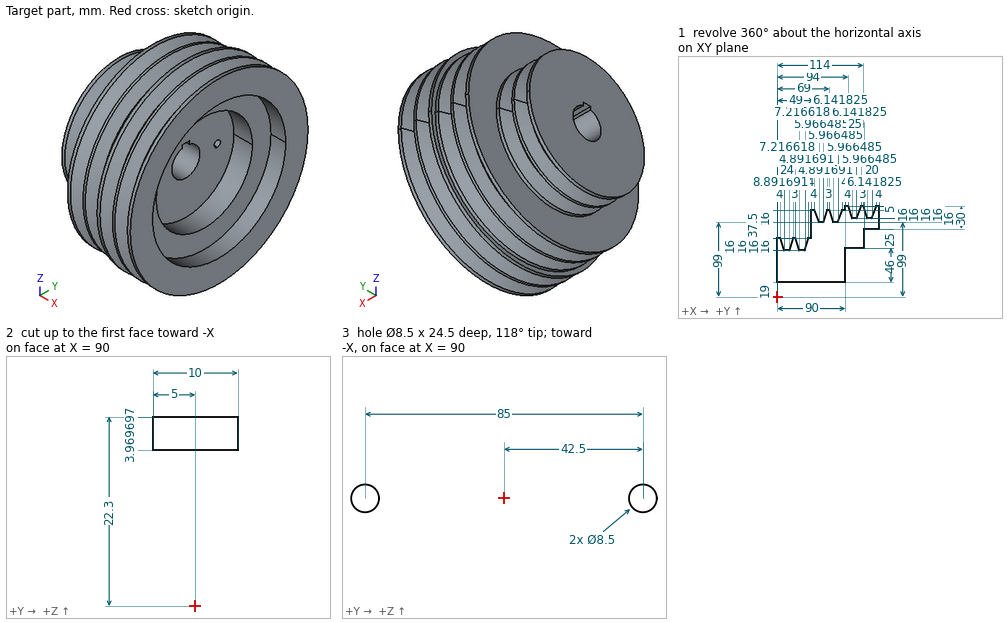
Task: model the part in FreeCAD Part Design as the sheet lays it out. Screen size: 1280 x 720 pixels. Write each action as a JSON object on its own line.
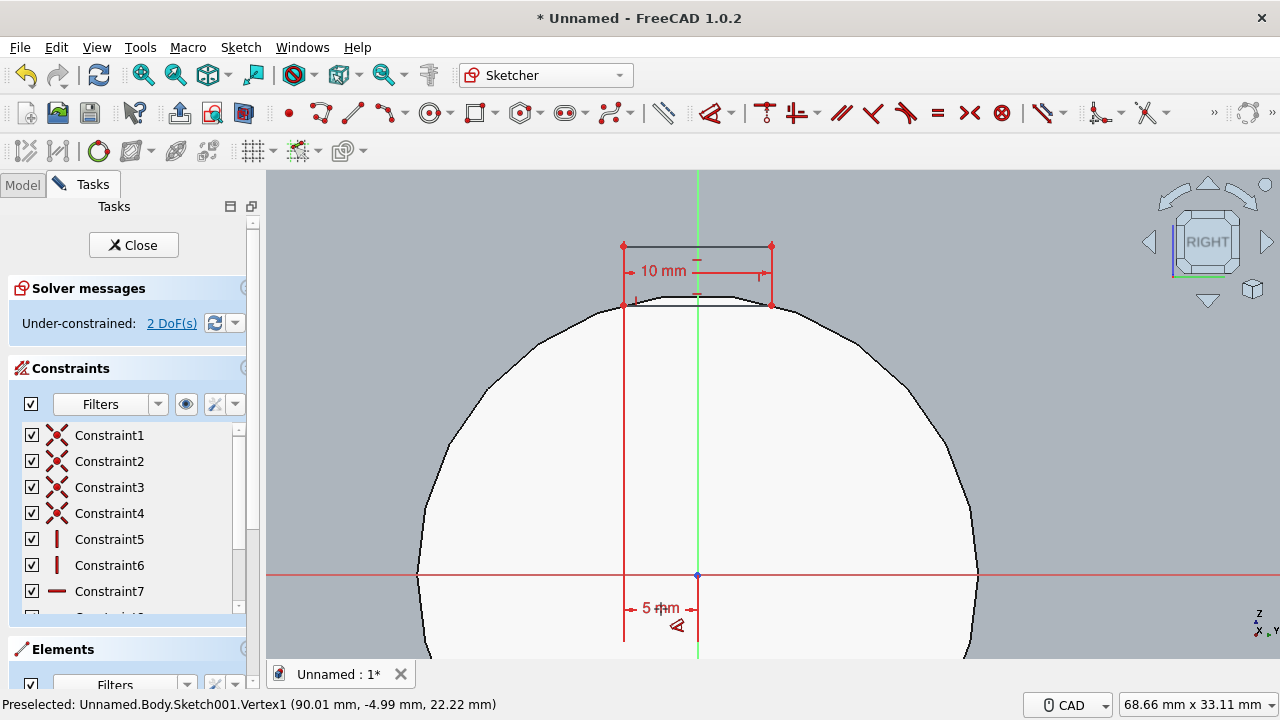
{"action": "left_click", "coordinate": [624, 247]}
{"action": "left_click", "coordinate": [590, 411]}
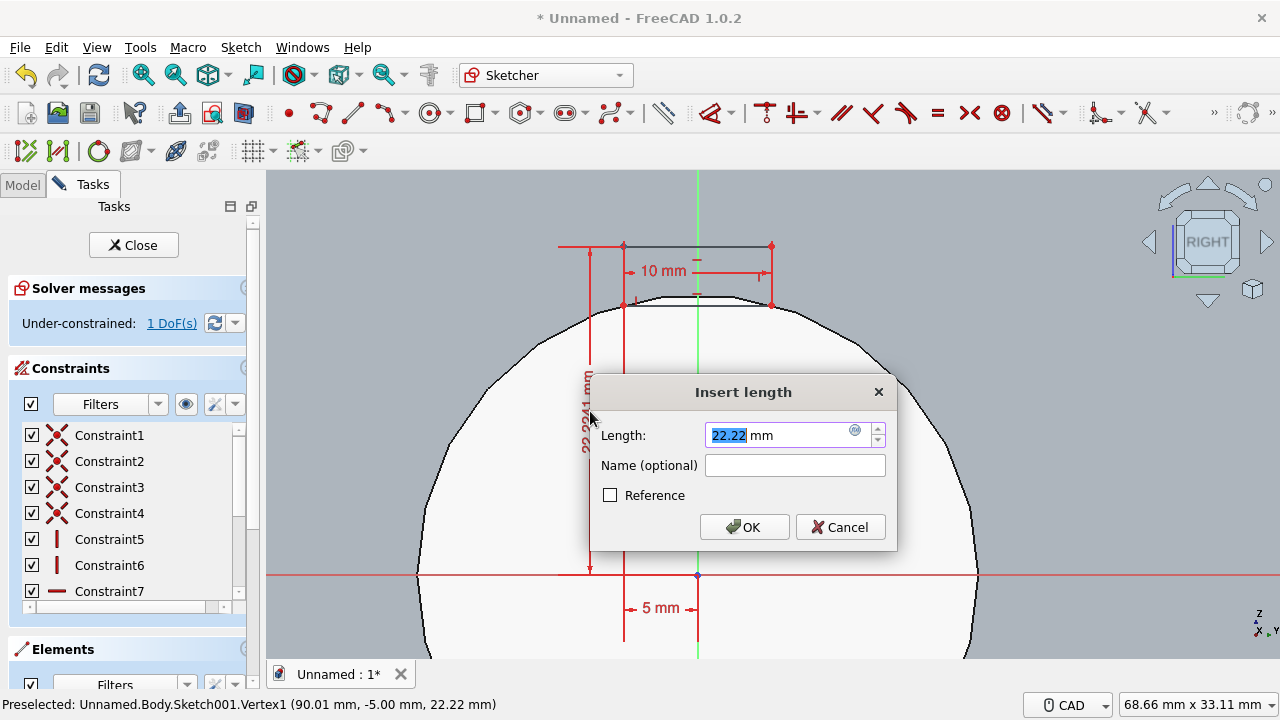
{"action": "type", "text": "22.3"}
{"action": "key", "text": "Return"}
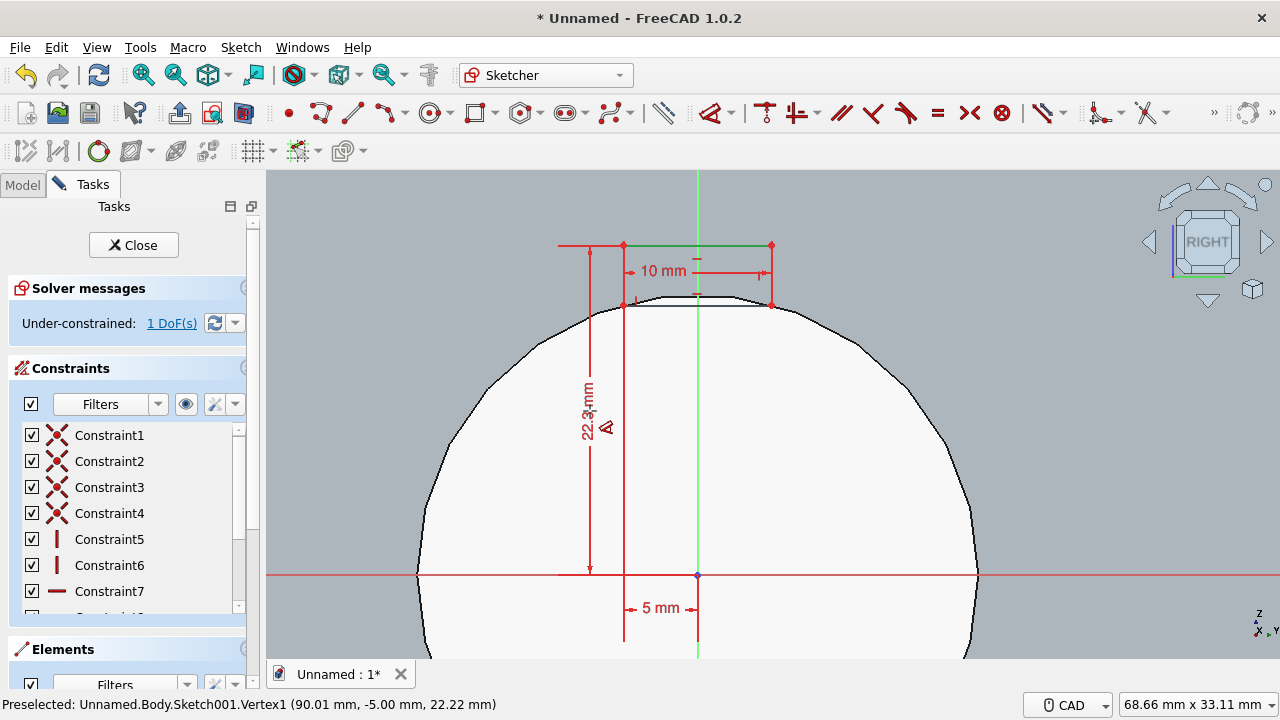
{"action": "left_click", "coordinate": [624, 264]}
{"action": "left_click", "coordinate": [590, 276]}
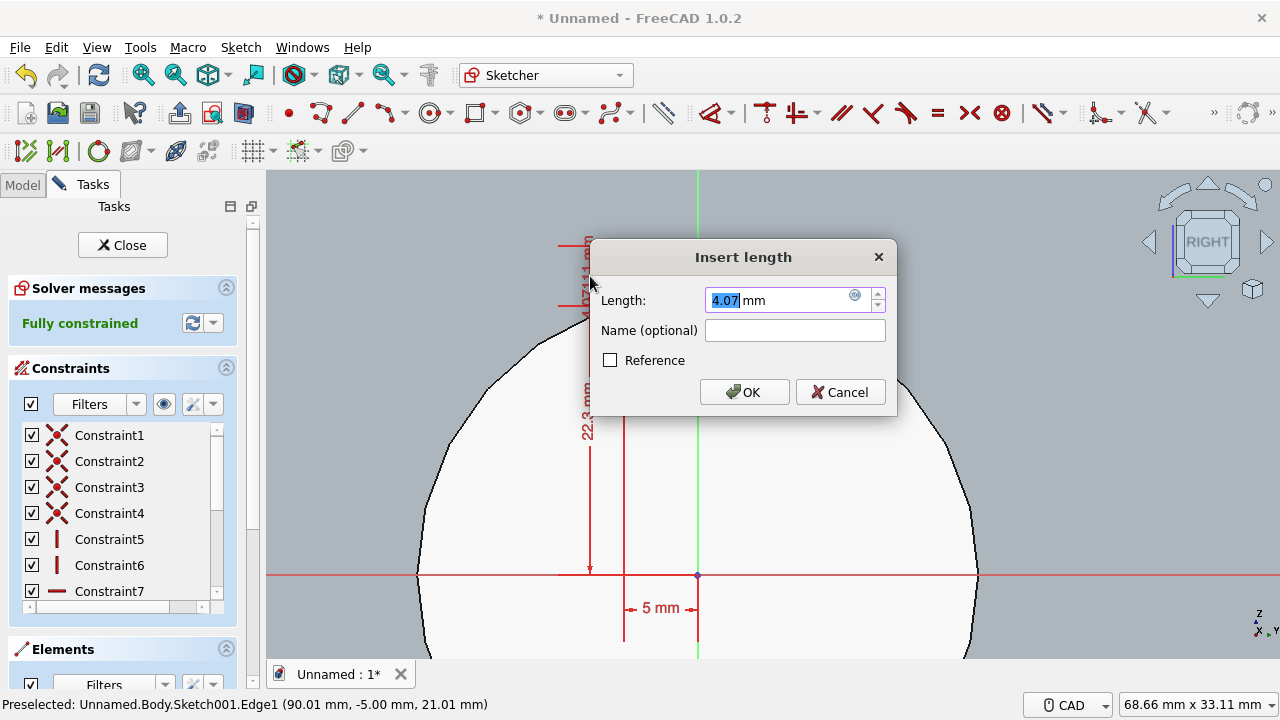
{"action": "type", "text": "3.969697"}
{"action": "key", "text": "Return"}
{"action": "key", "text": "Escape"}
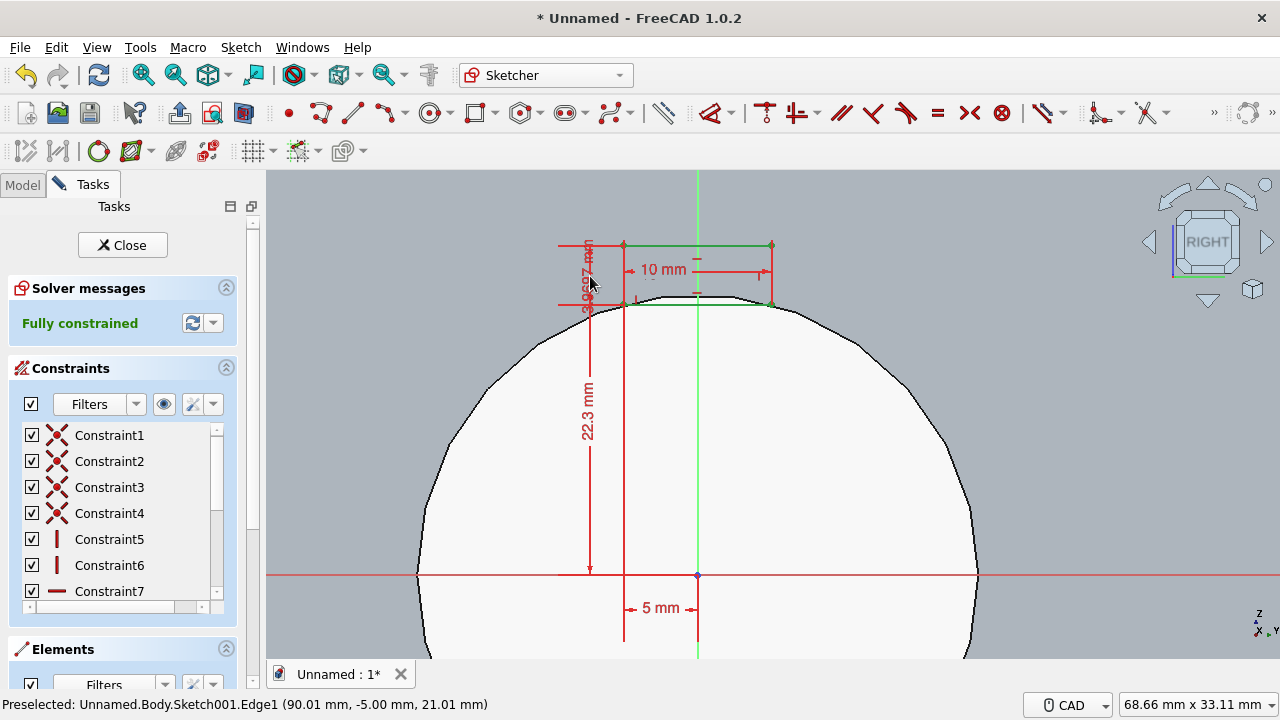
{"action": "left_click", "coordinate": [123, 245]}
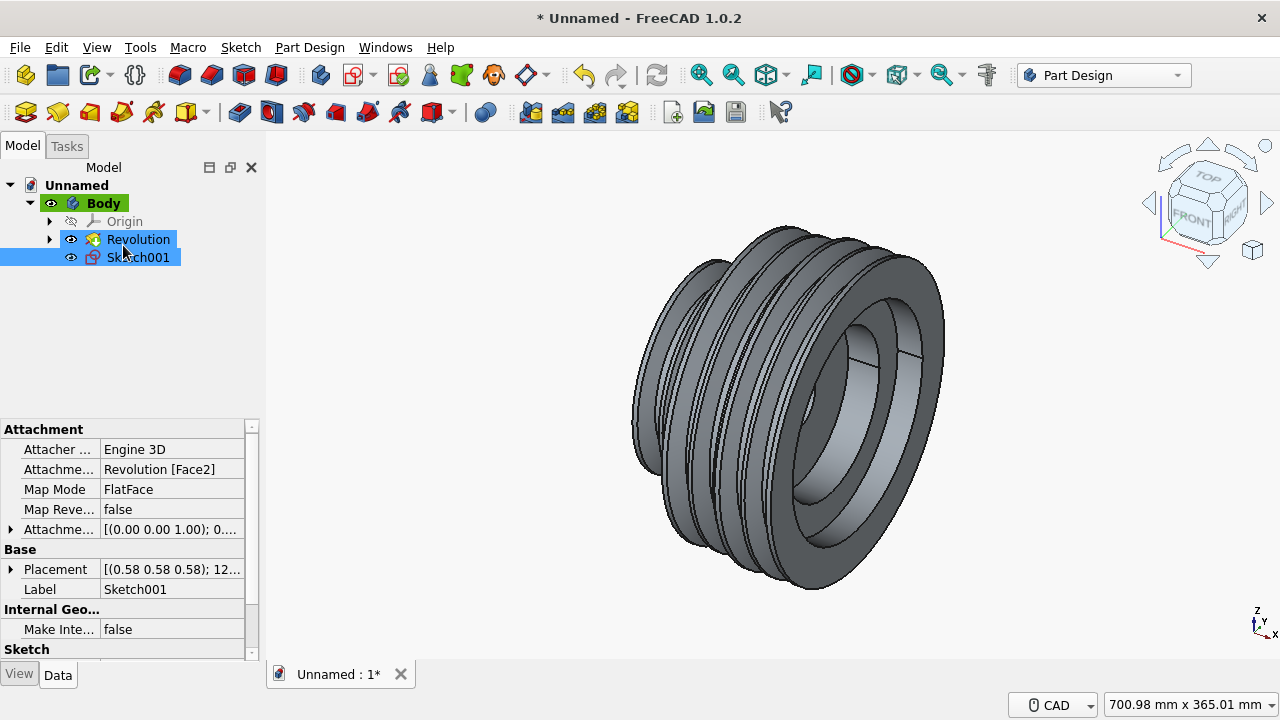
{"action": "left_click", "coordinate": [240, 112]}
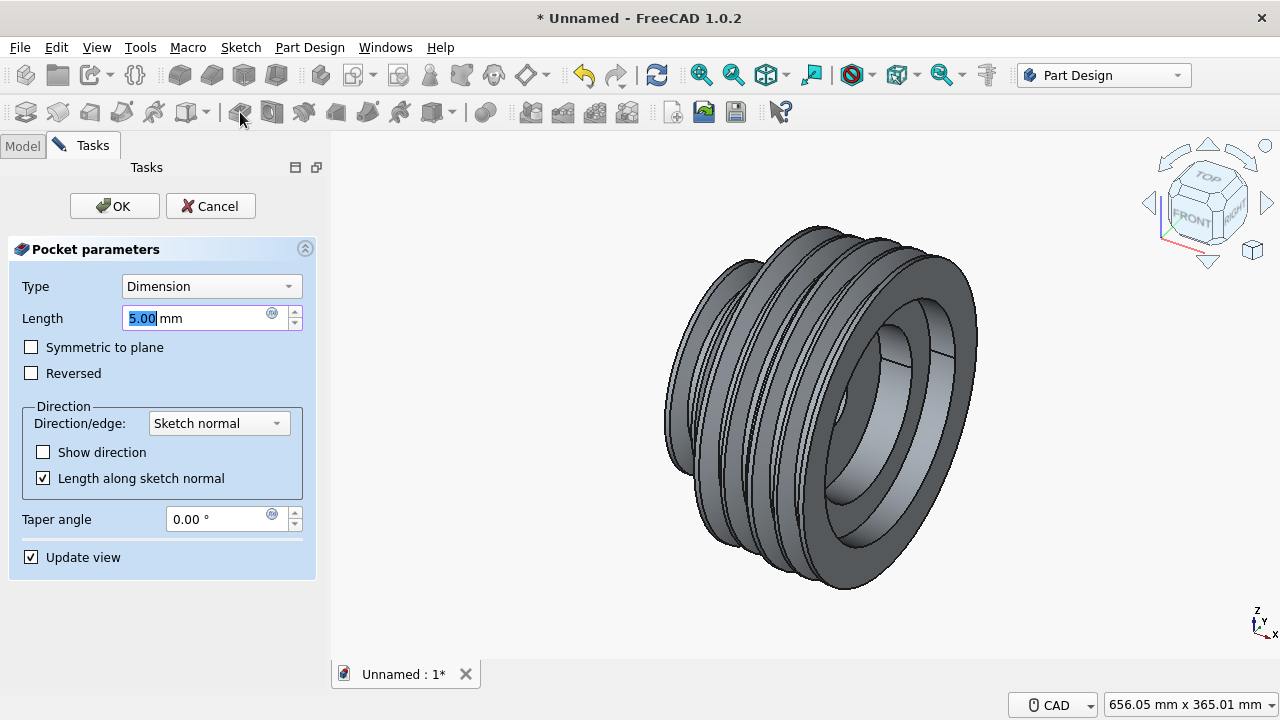
{"action": "left_click", "coordinate": [212, 286]}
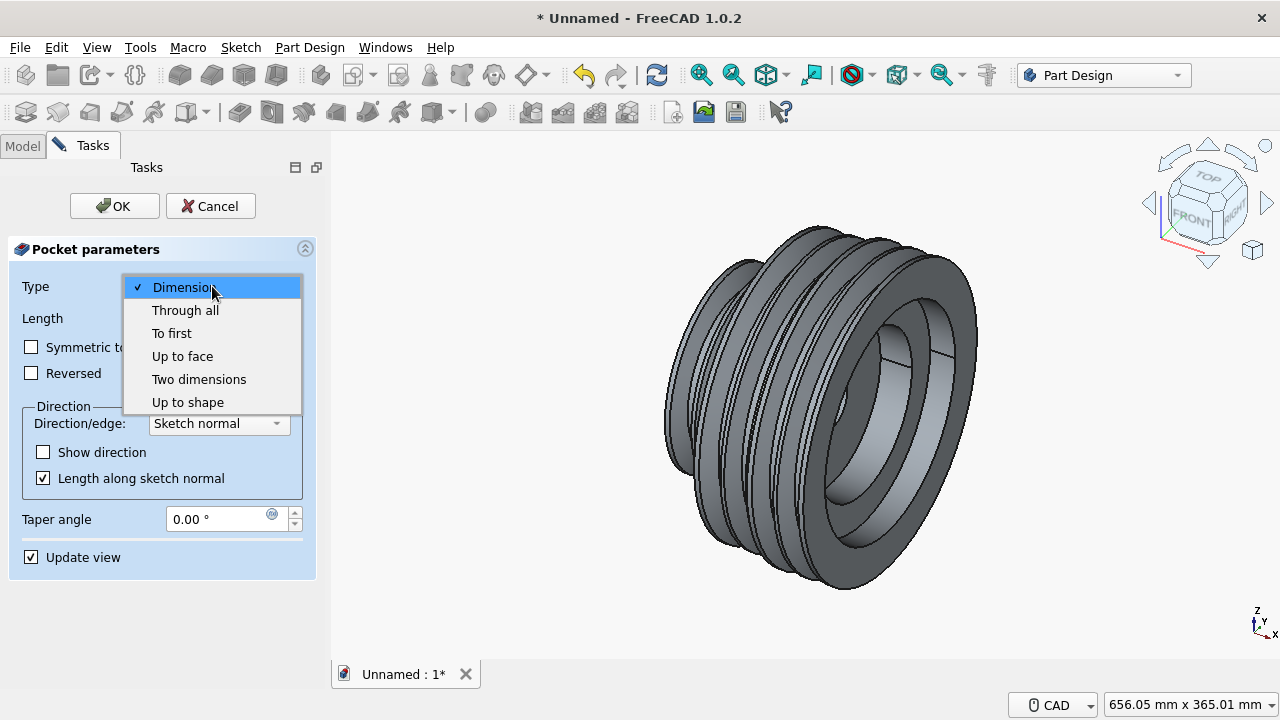
{"action": "left_click", "coordinate": [212, 334]}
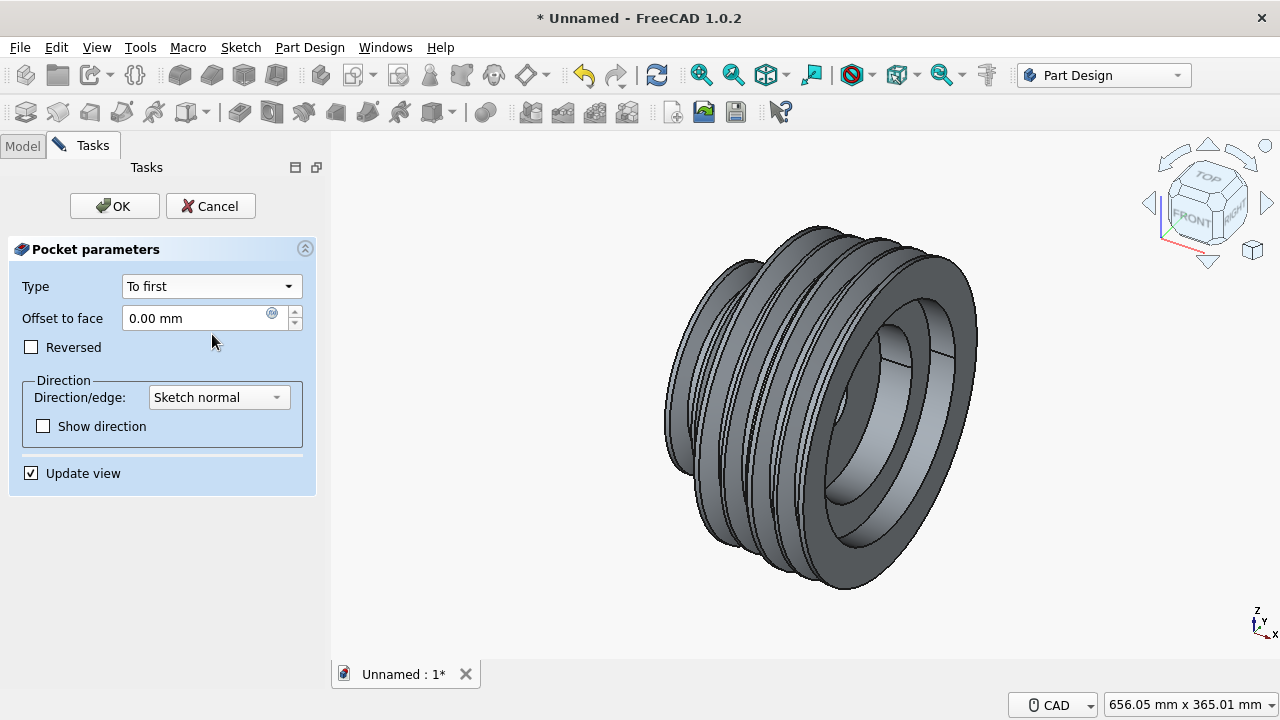
{"action": "left_click", "coordinate": [115, 206]}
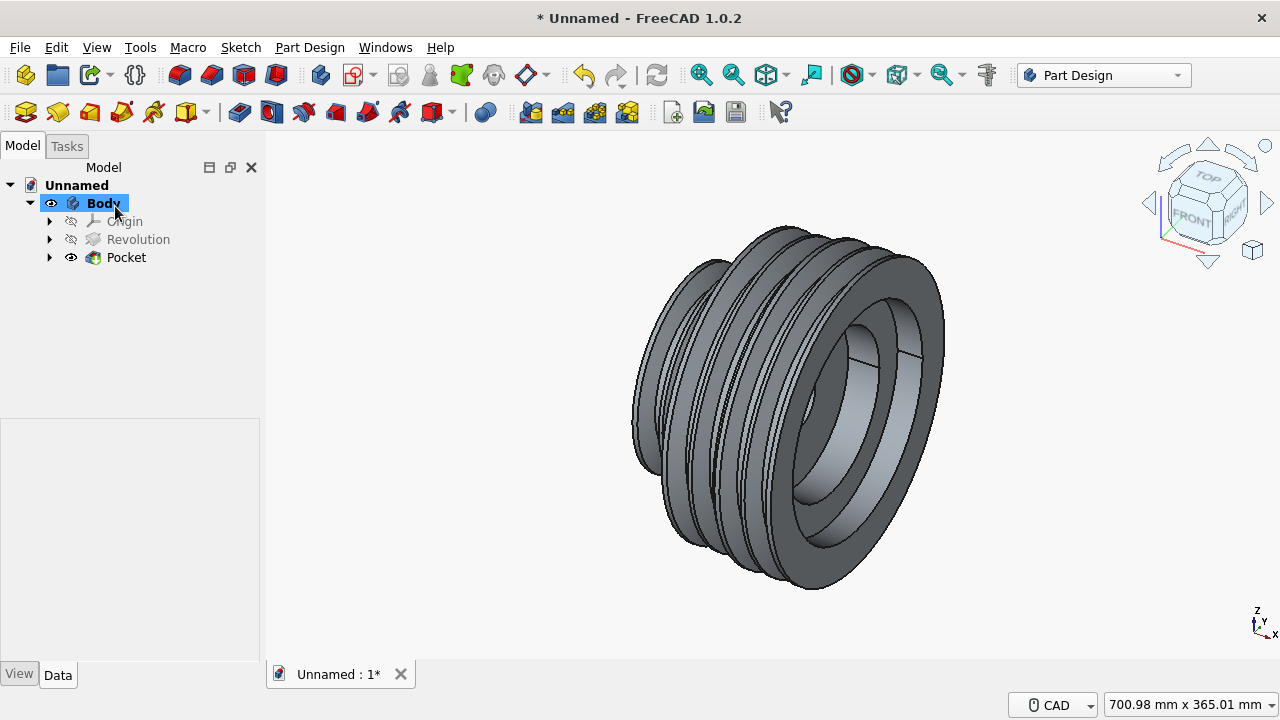
{"action": "left_click", "coordinate": [828, 399]}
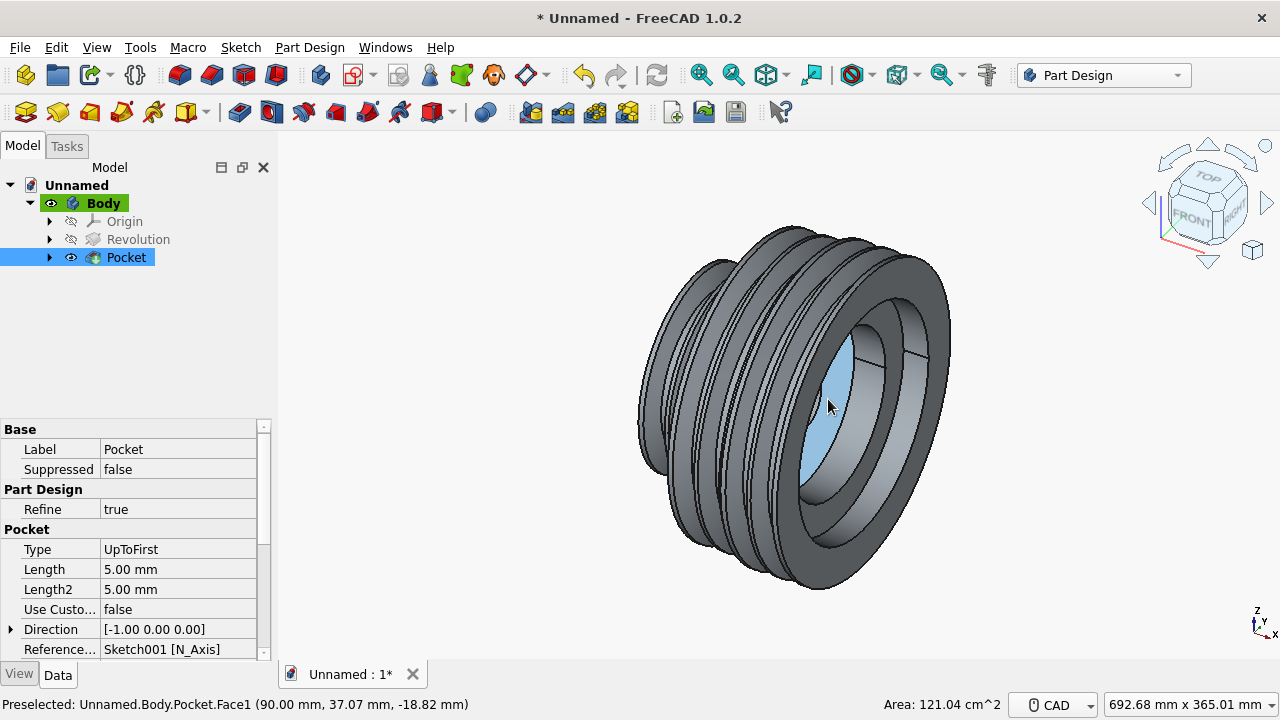
{"action": "left_click", "coordinate": [354, 76]}